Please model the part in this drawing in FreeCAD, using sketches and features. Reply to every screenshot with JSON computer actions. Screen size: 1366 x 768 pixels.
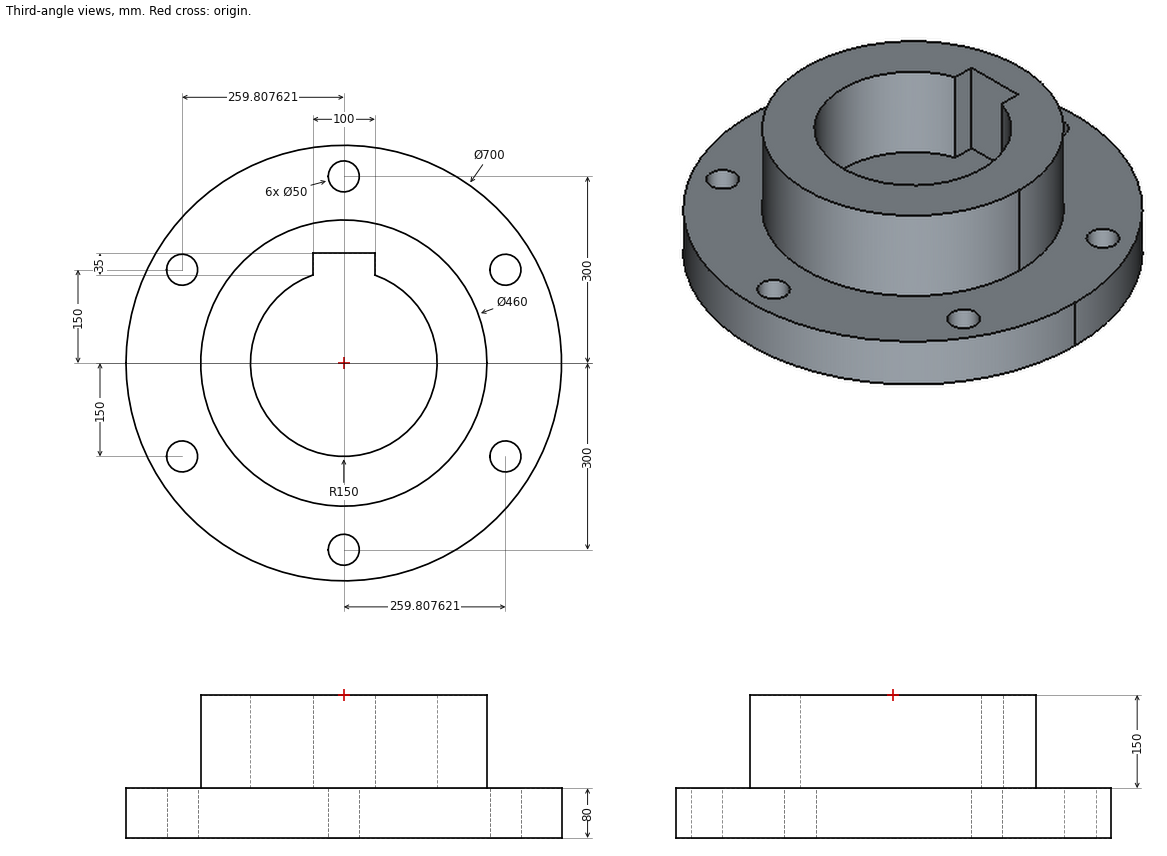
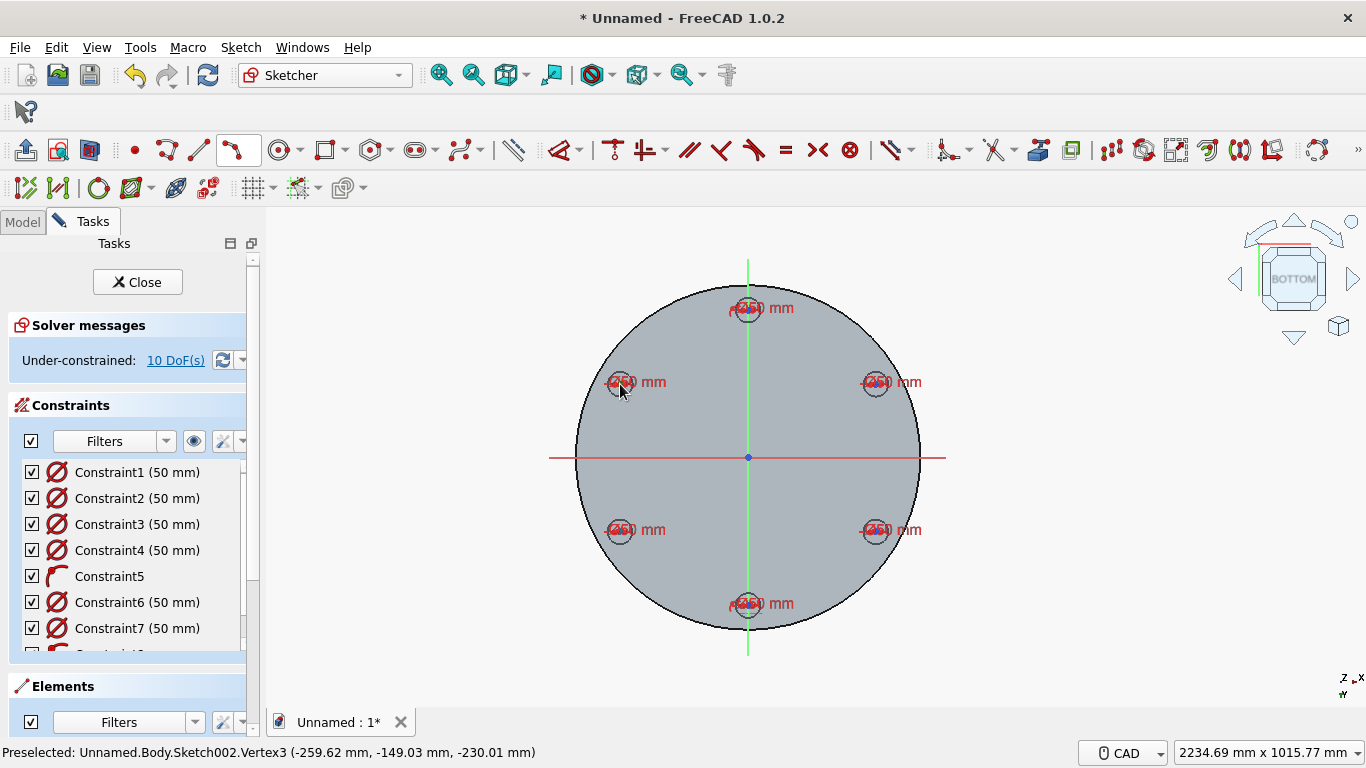
{"action": "left_click", "coordinate": [668, 150]}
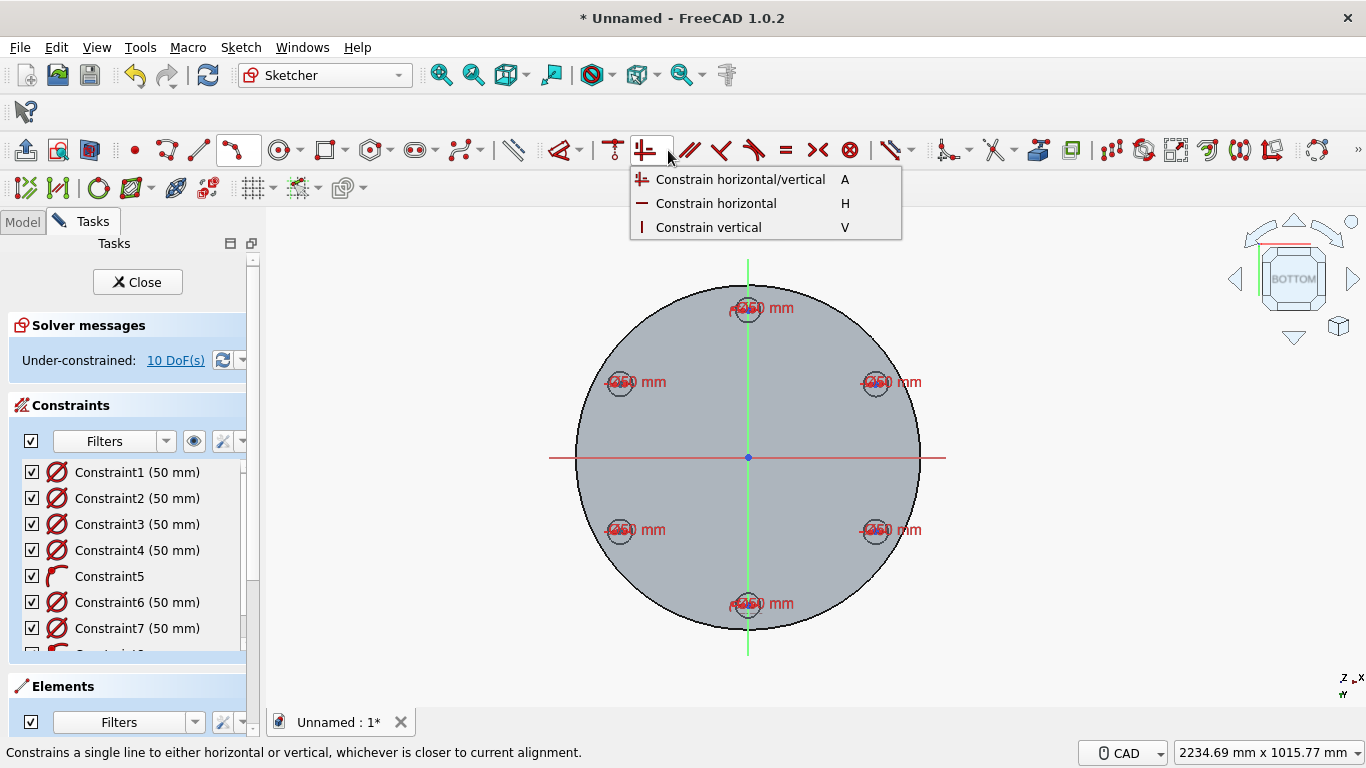
{"action": "left_click", "coordinate": [766, 227]}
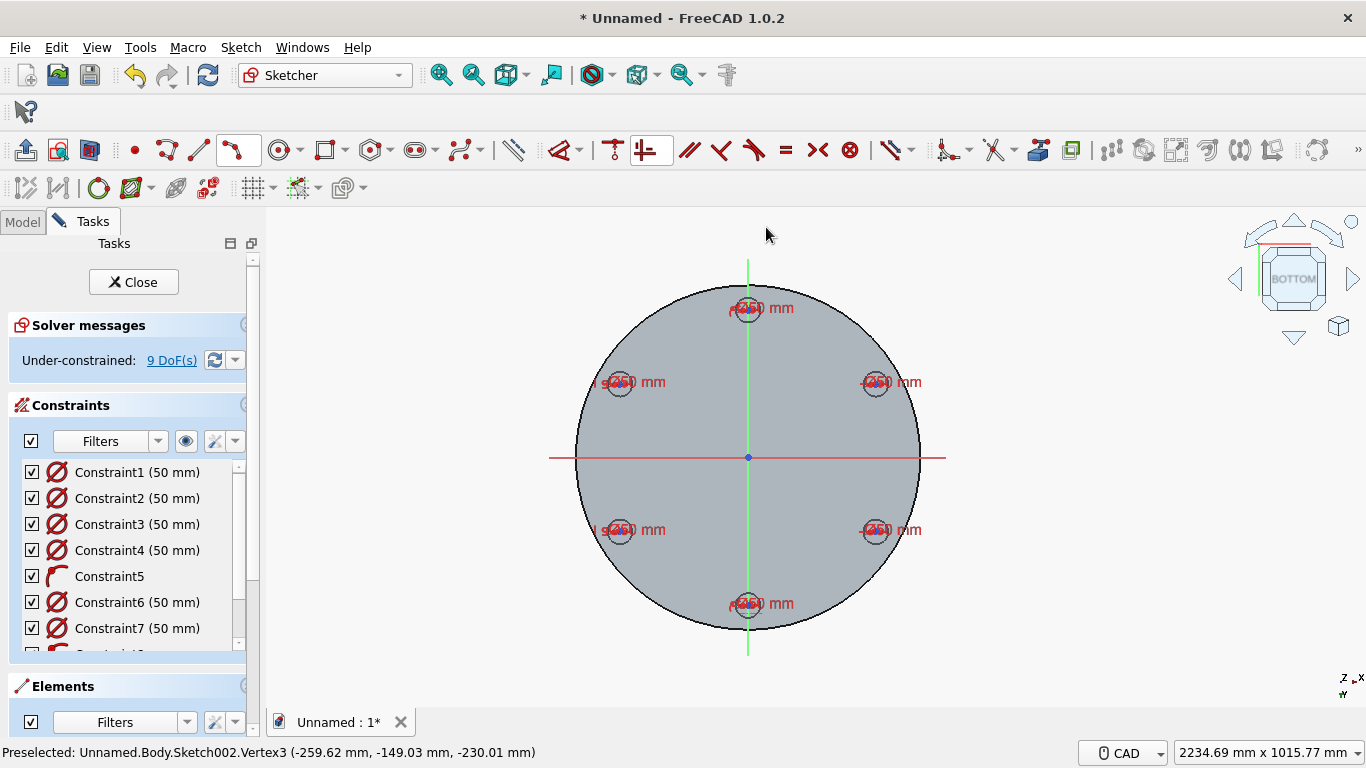
{"action": "left_click", "coordinate": [620, 384]}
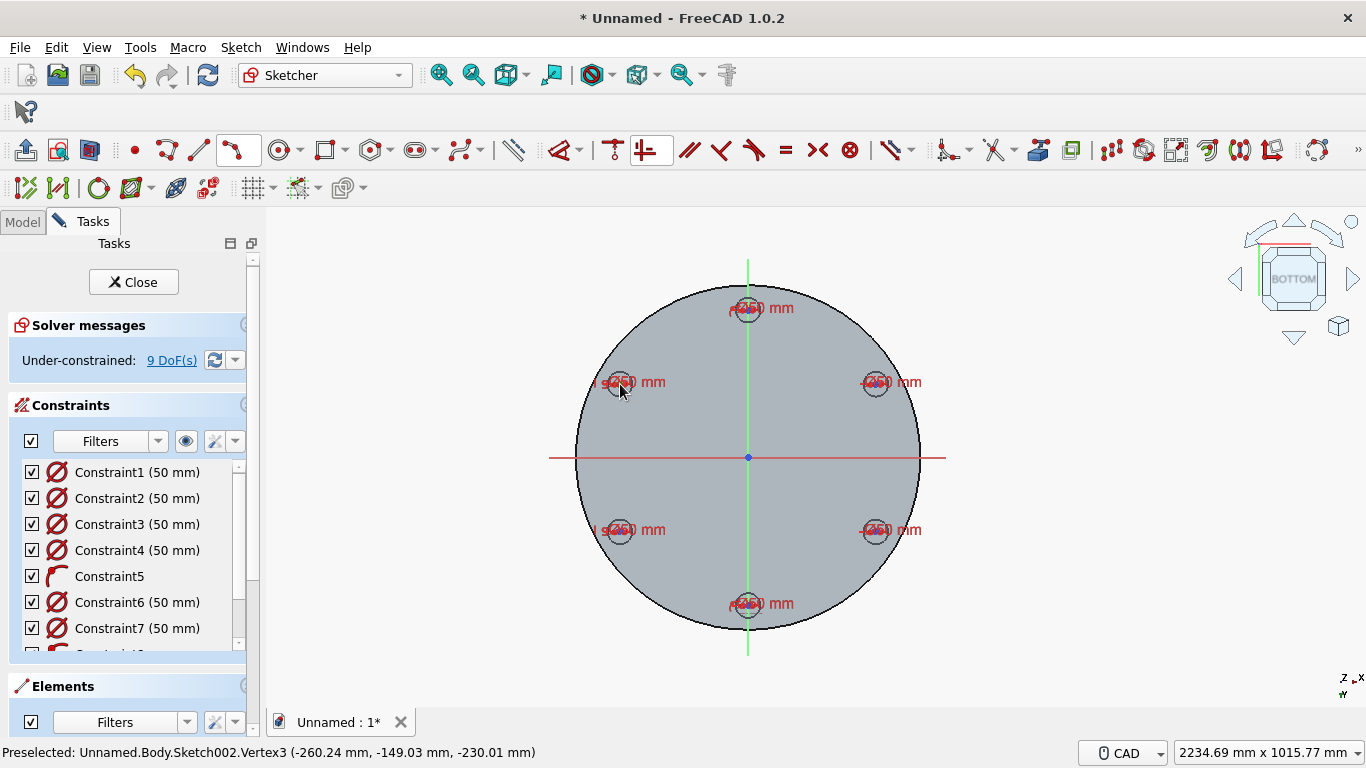
{"action": "left_click", "coordinate": [876, 384]}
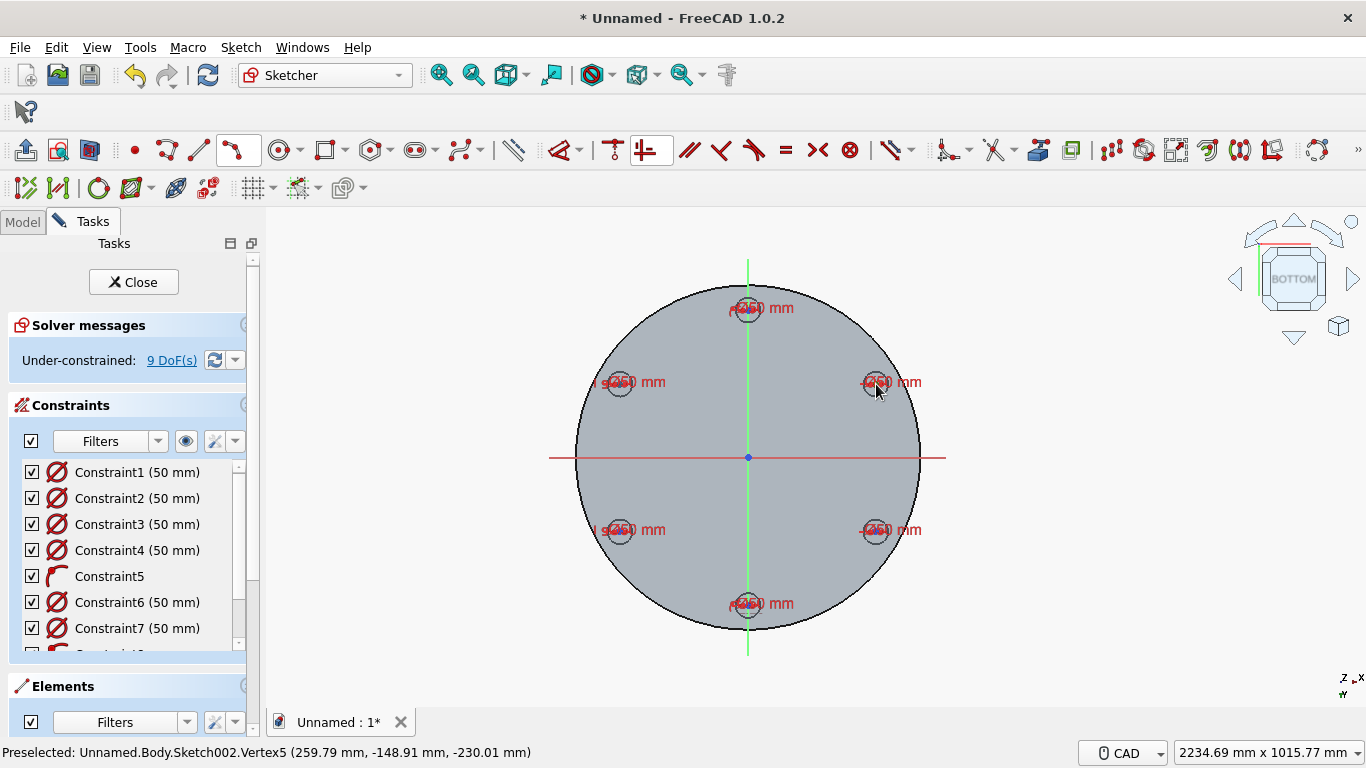
{"action": "key", "text": "h"}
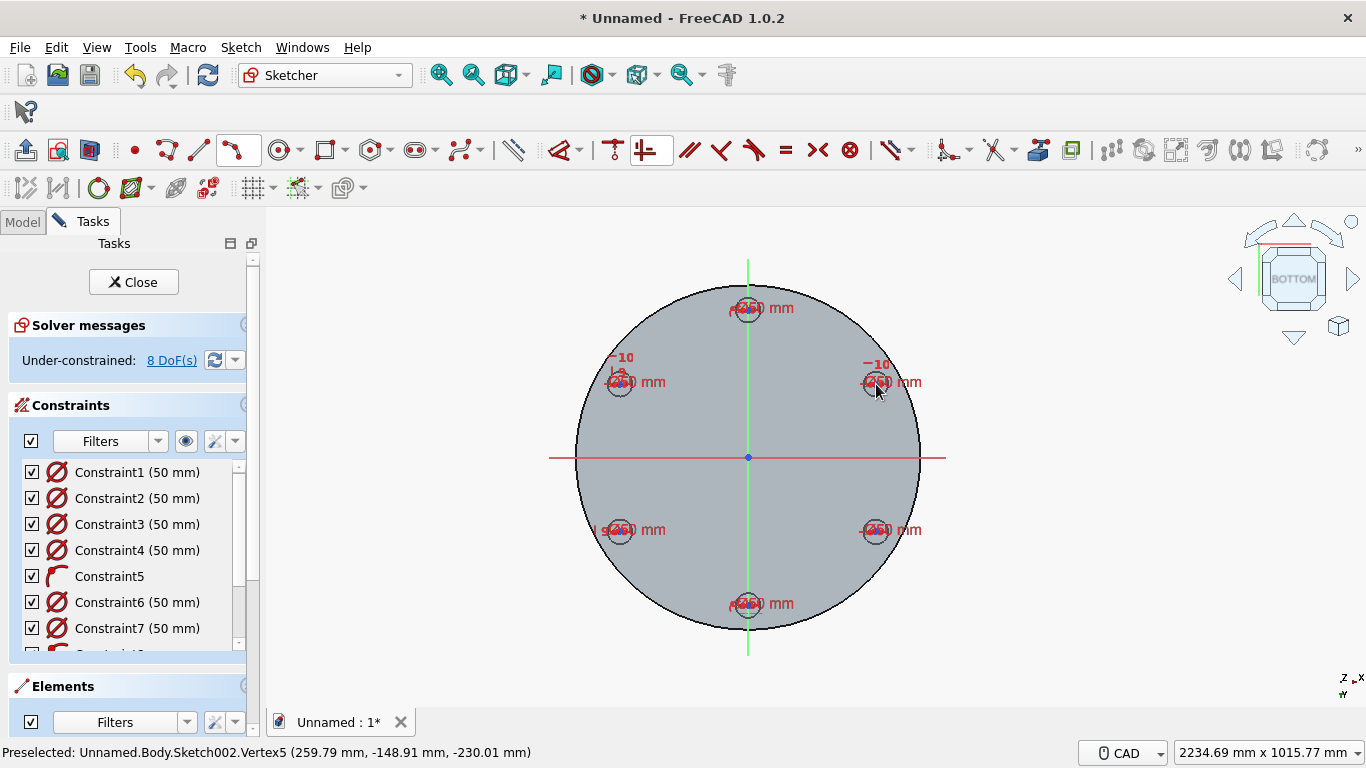
{"action": "left_click", "coordinate": [876, 384]}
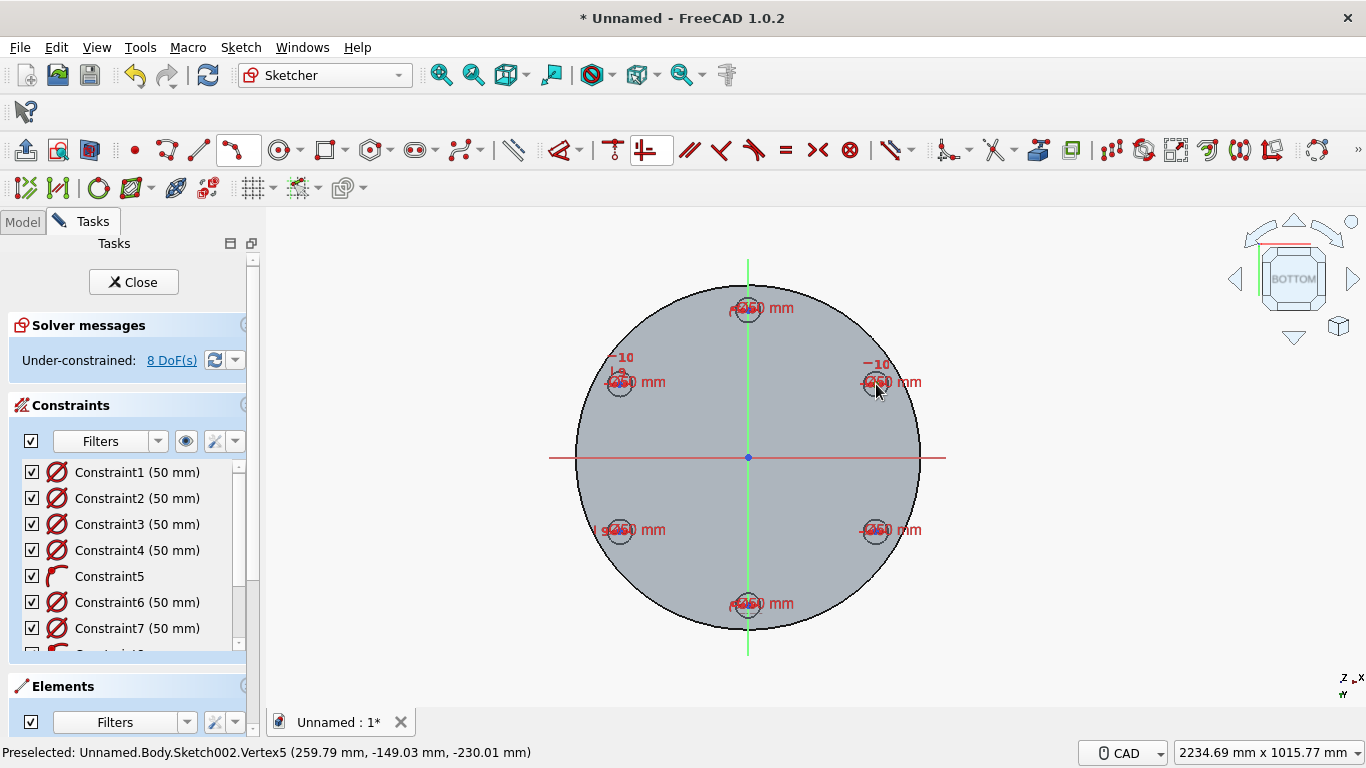
{"action": "left_click", "coordinate": [876, 532]}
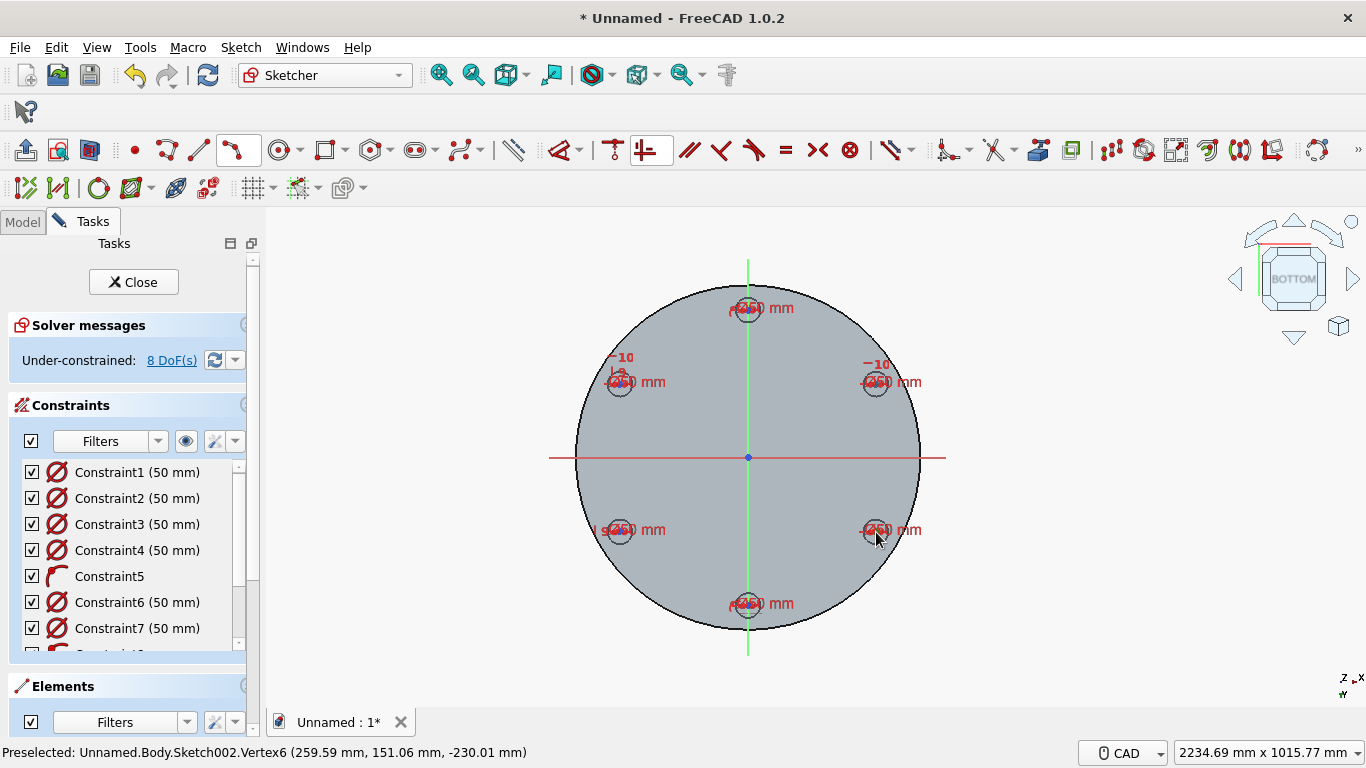
{"action": "key", "text": "v"}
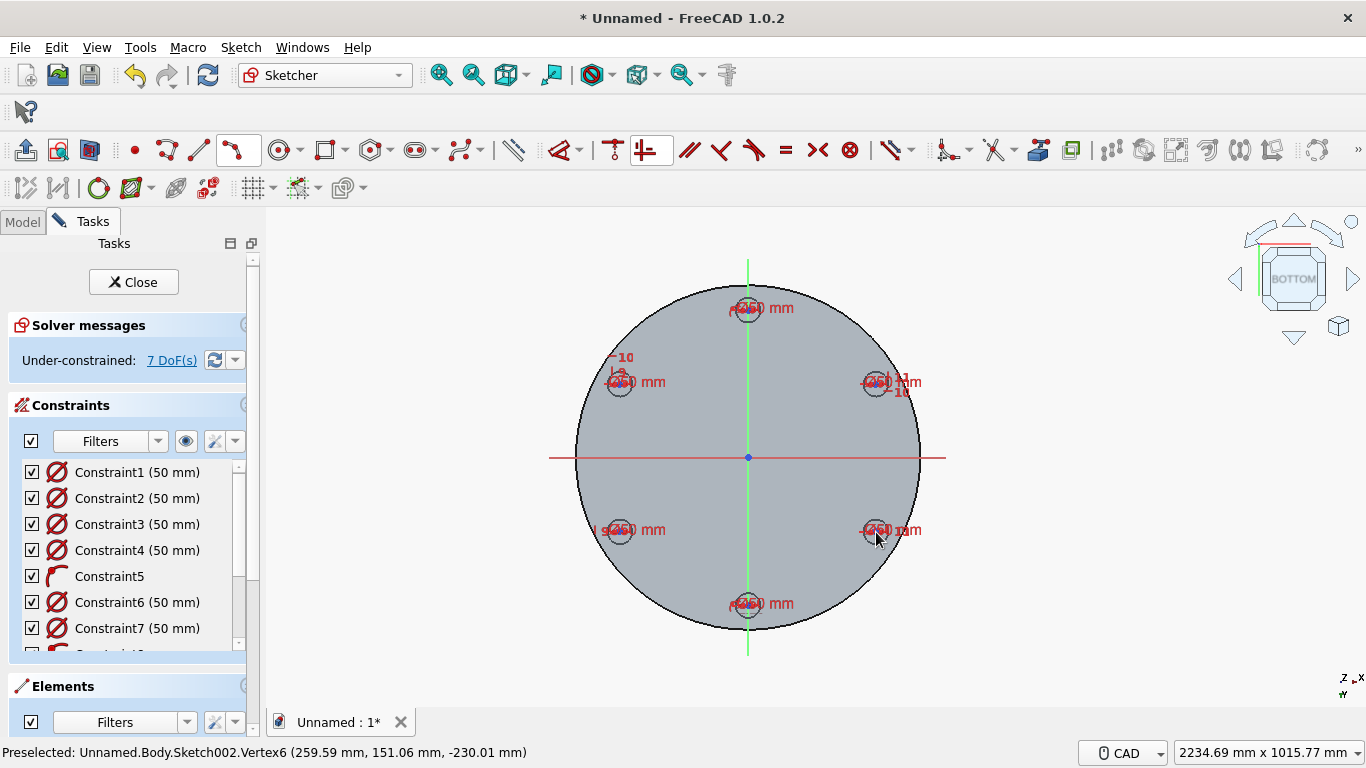
{"action": "left_click", "coordinate": [620, 532]}